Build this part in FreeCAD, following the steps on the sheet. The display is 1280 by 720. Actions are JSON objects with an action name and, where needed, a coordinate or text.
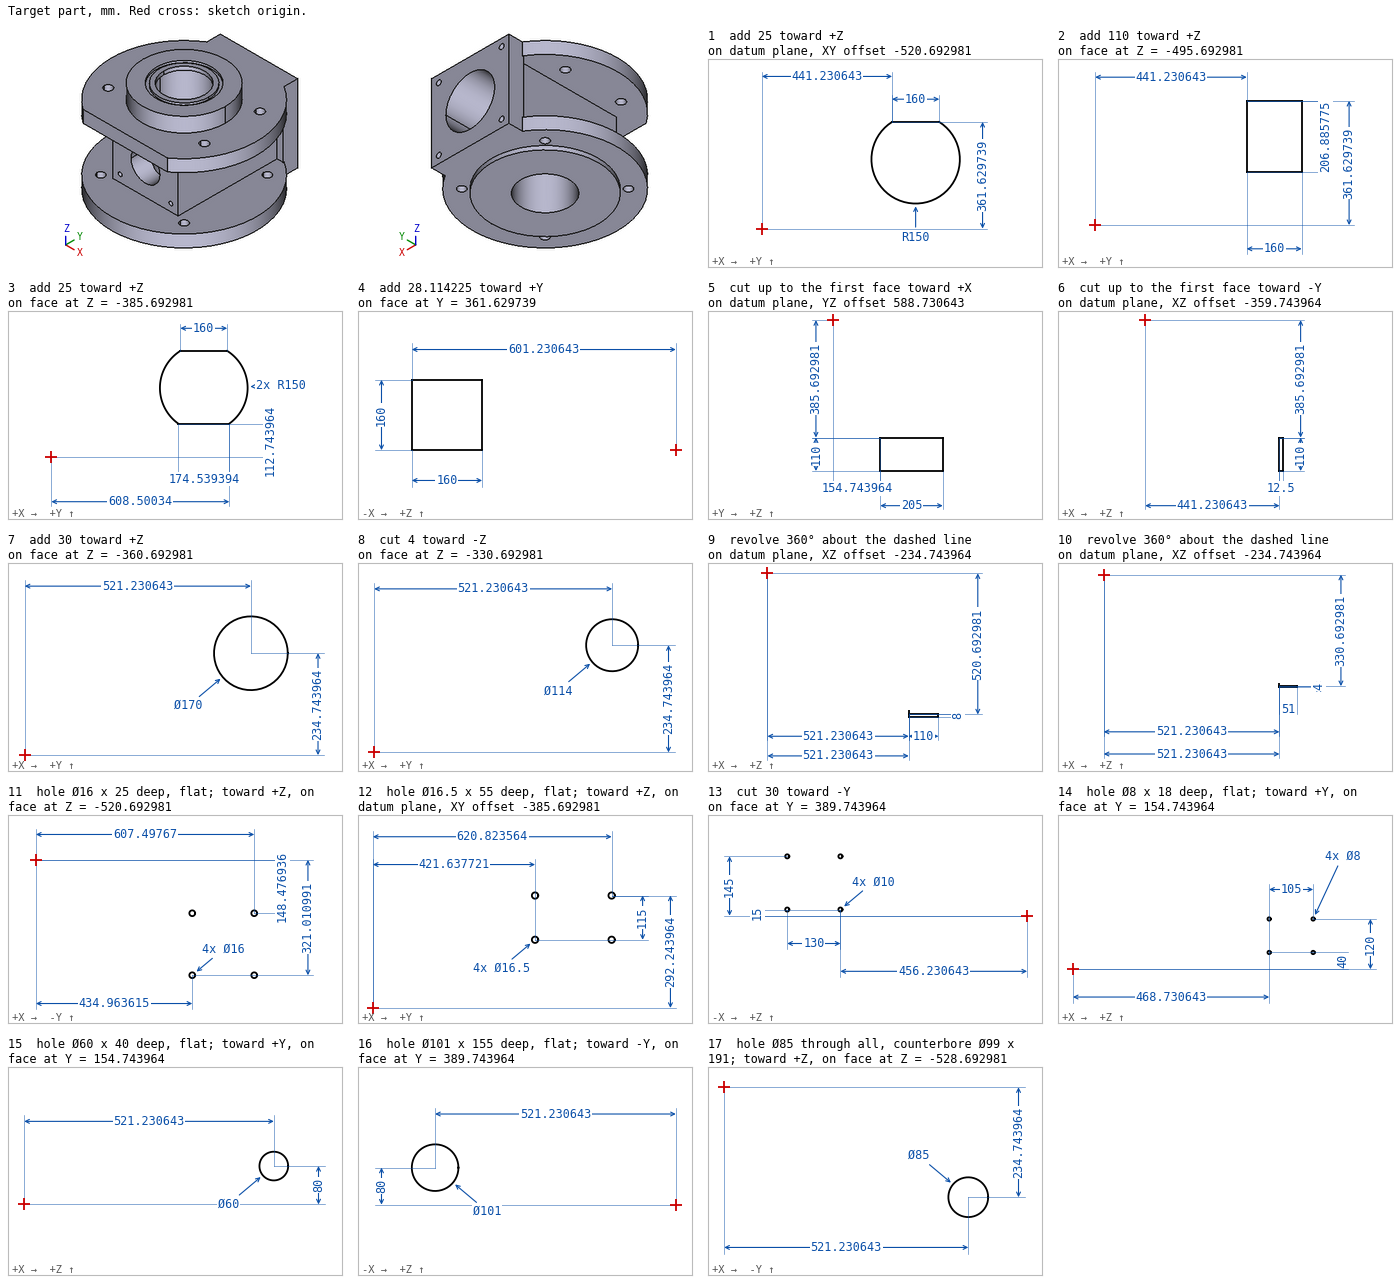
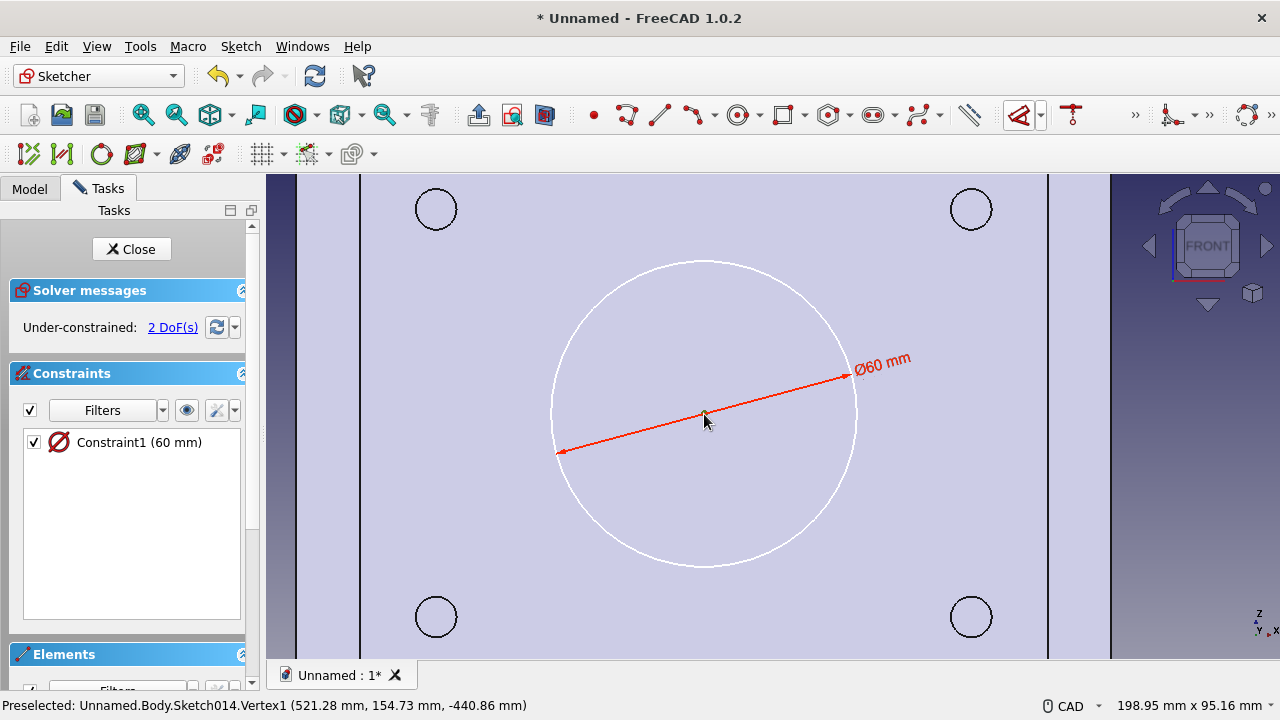
{"action": "key", "text": "i"}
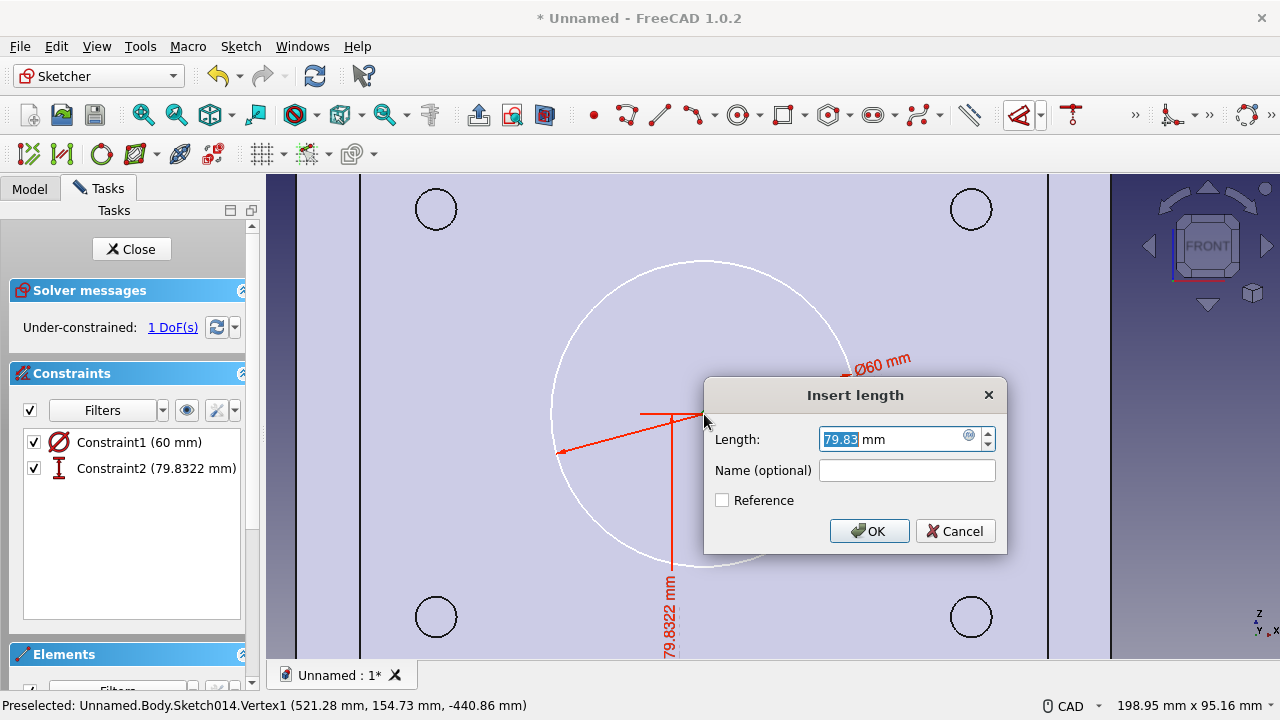
{"action": "type", "text": "80"}
{"action": "key", "text": "Return"}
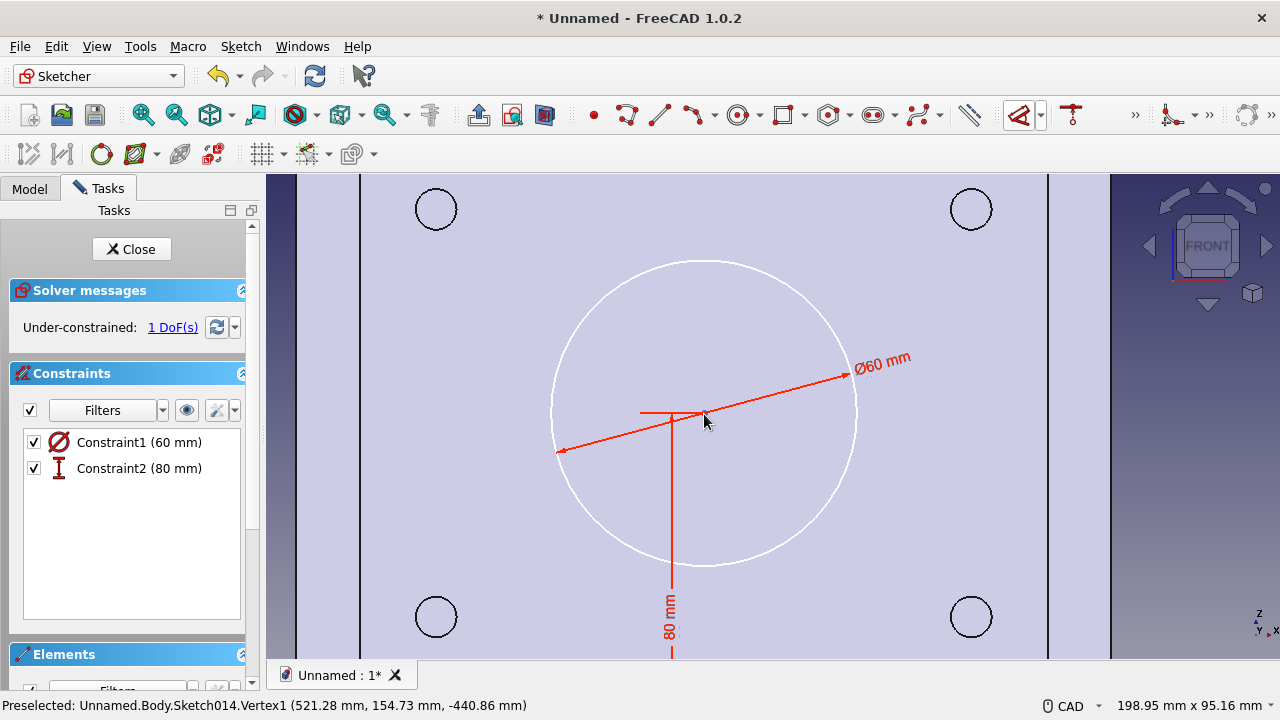
{"action": "left_click", "coordinate": [704, 413]}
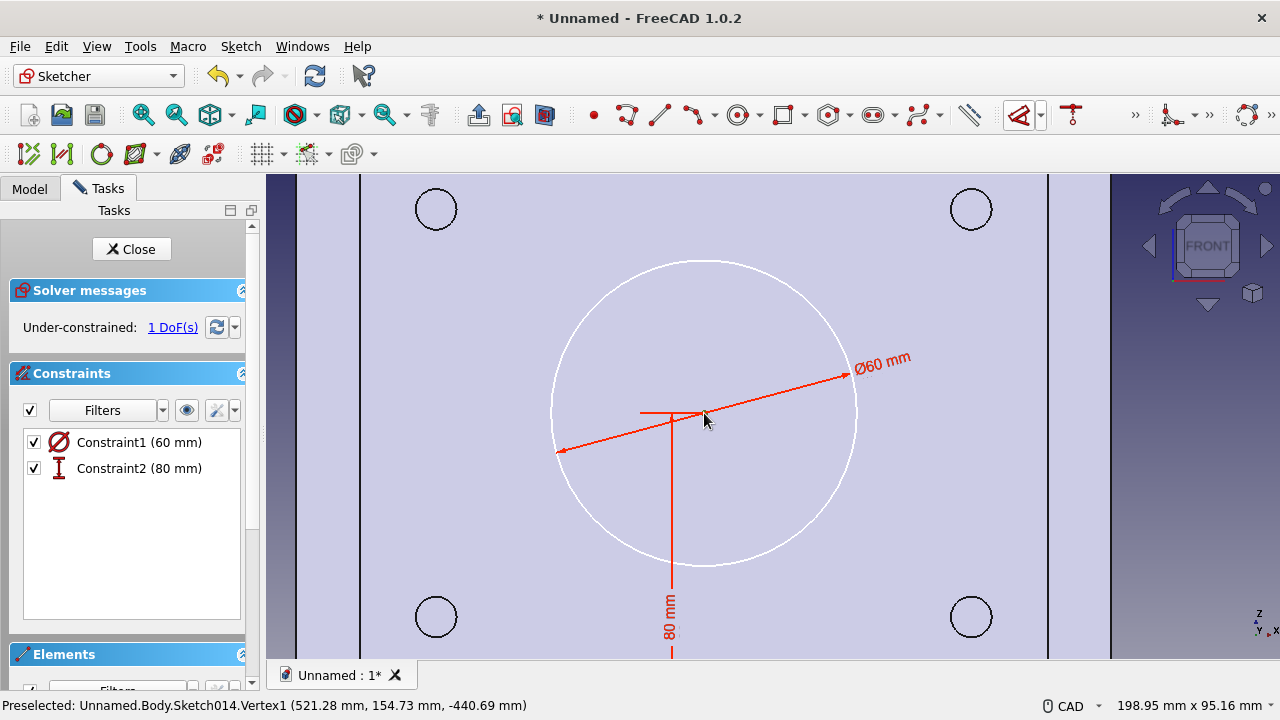
{"action": "left_click", "coordinate": [1040, 116]}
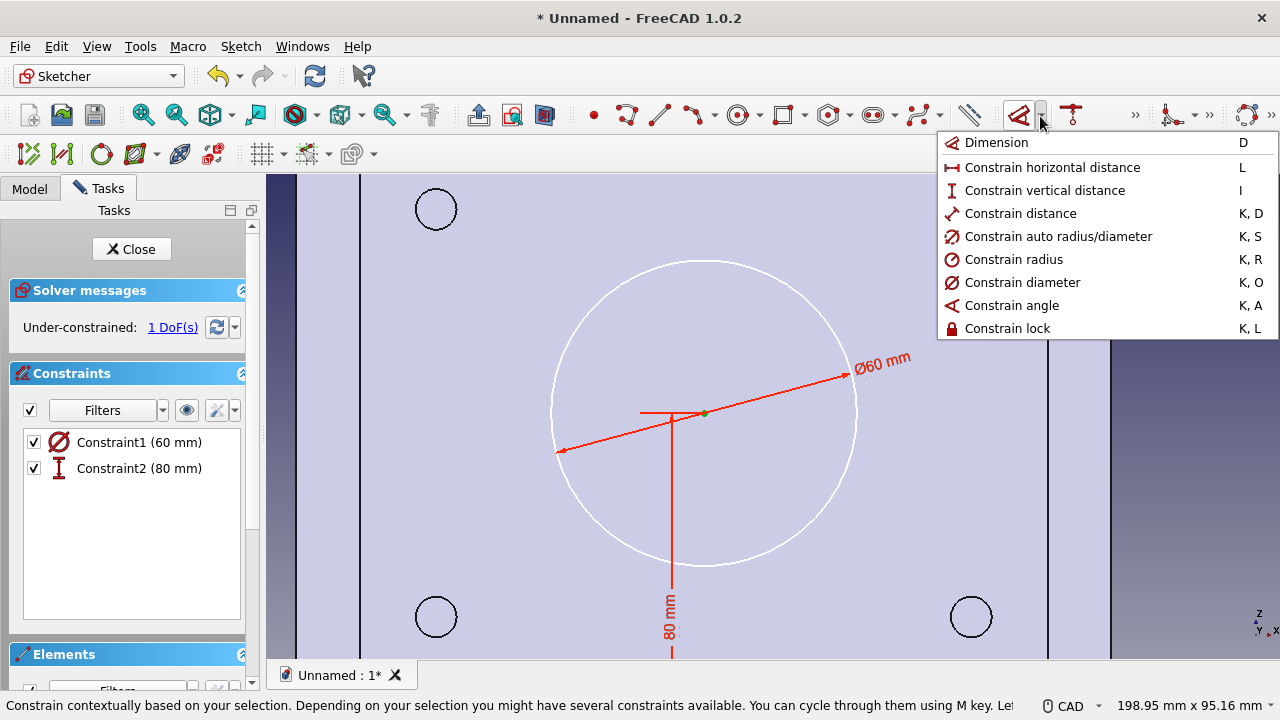
{"action": "left_click", "coordinate": [1108, 168]}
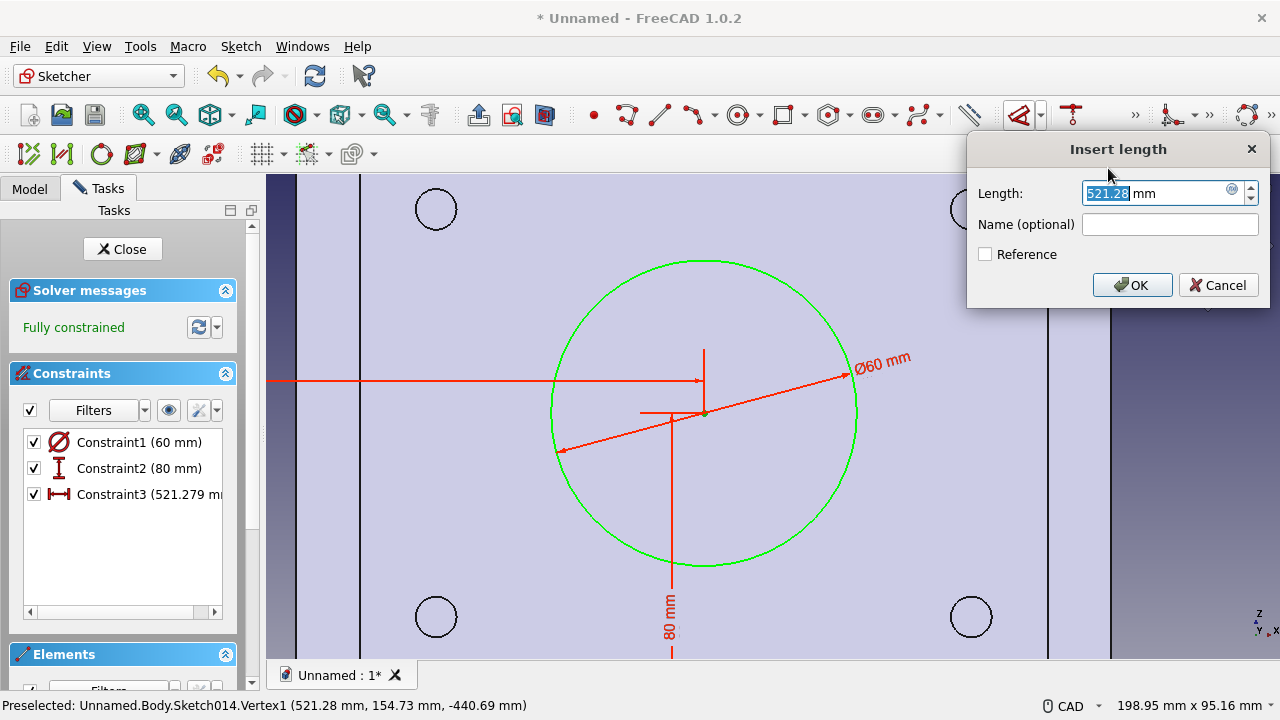
{"action": "type", "text": "521.230643"}
{"action": "key", "text": "Return"}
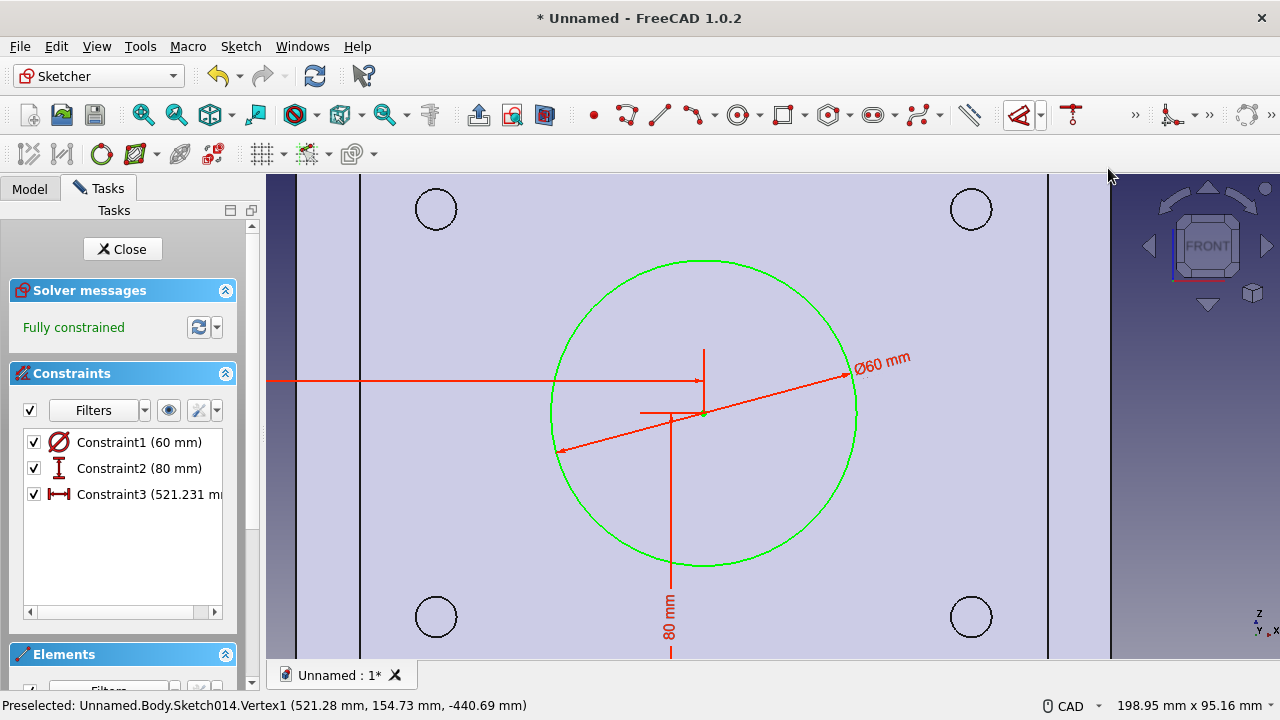
{"action": "left_click", "coordinate": [123, 249]}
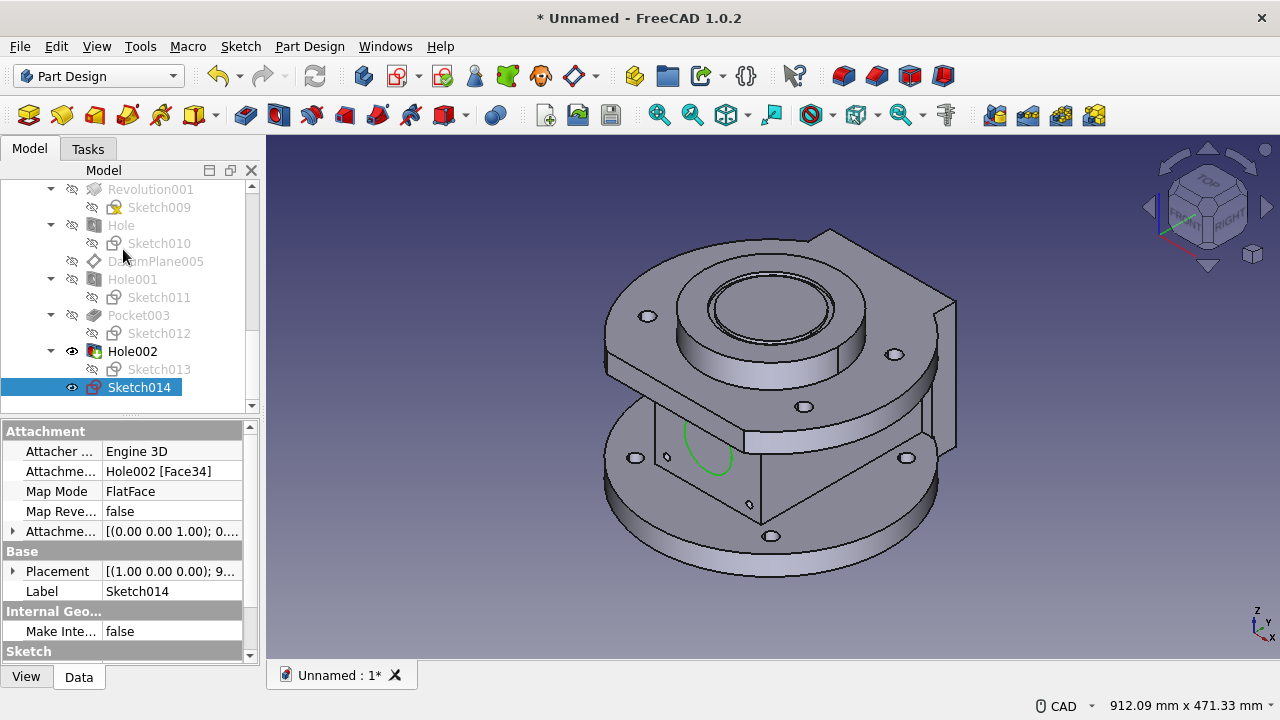
{"action": "left_click", "coordinate": [279, 116]}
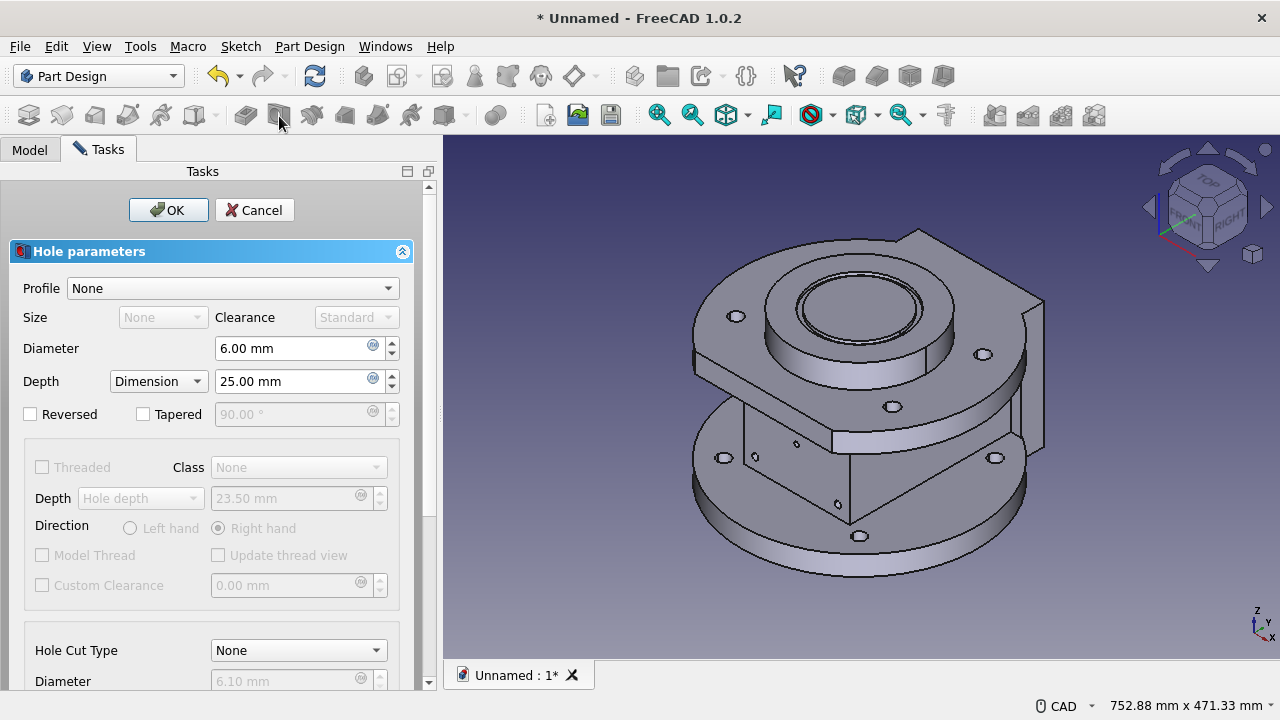
{"action": "triple_click", "coordinate": [300, 348]}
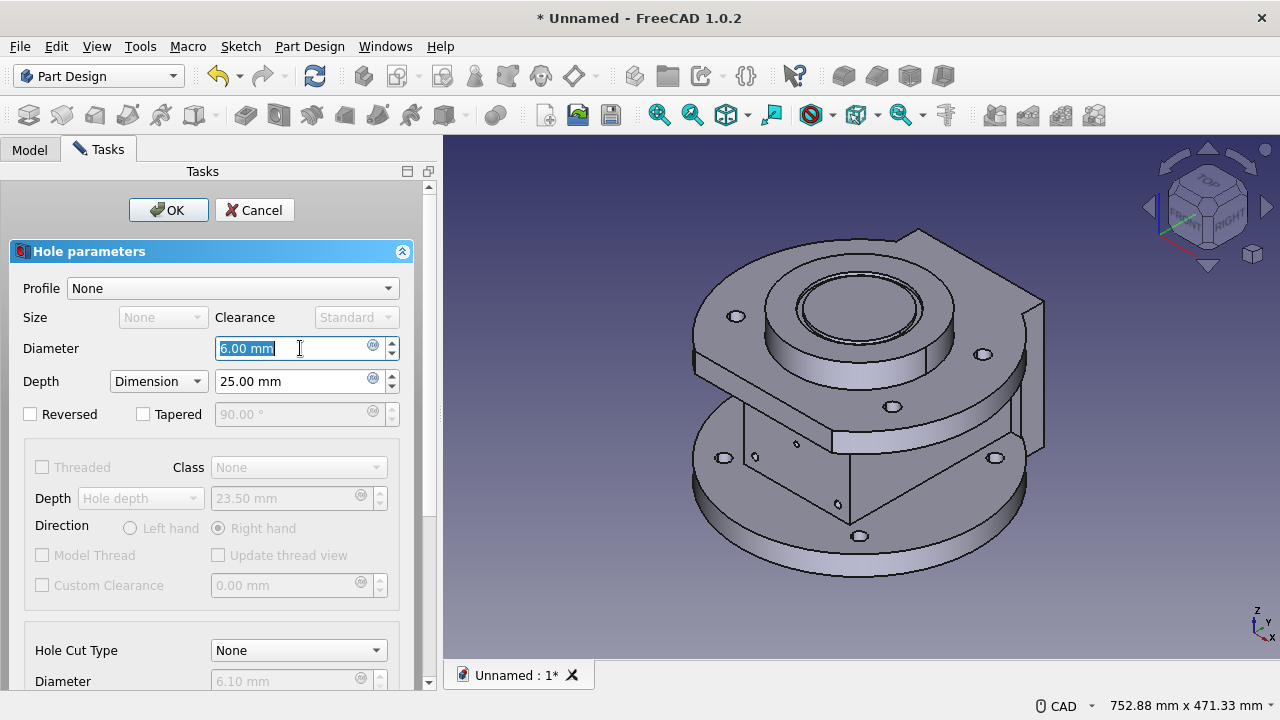
{"action": "type", "text": "60"}
{"action": "key", "text": "Tab"}